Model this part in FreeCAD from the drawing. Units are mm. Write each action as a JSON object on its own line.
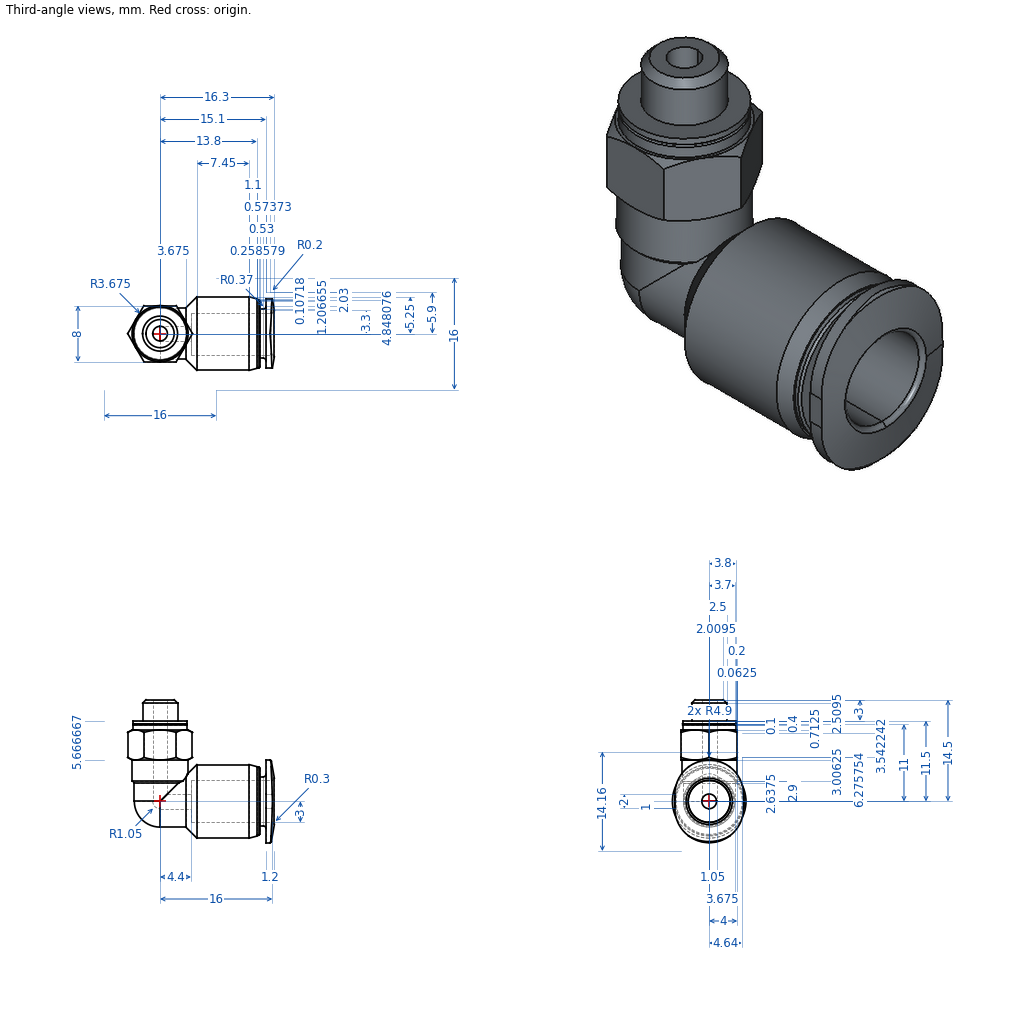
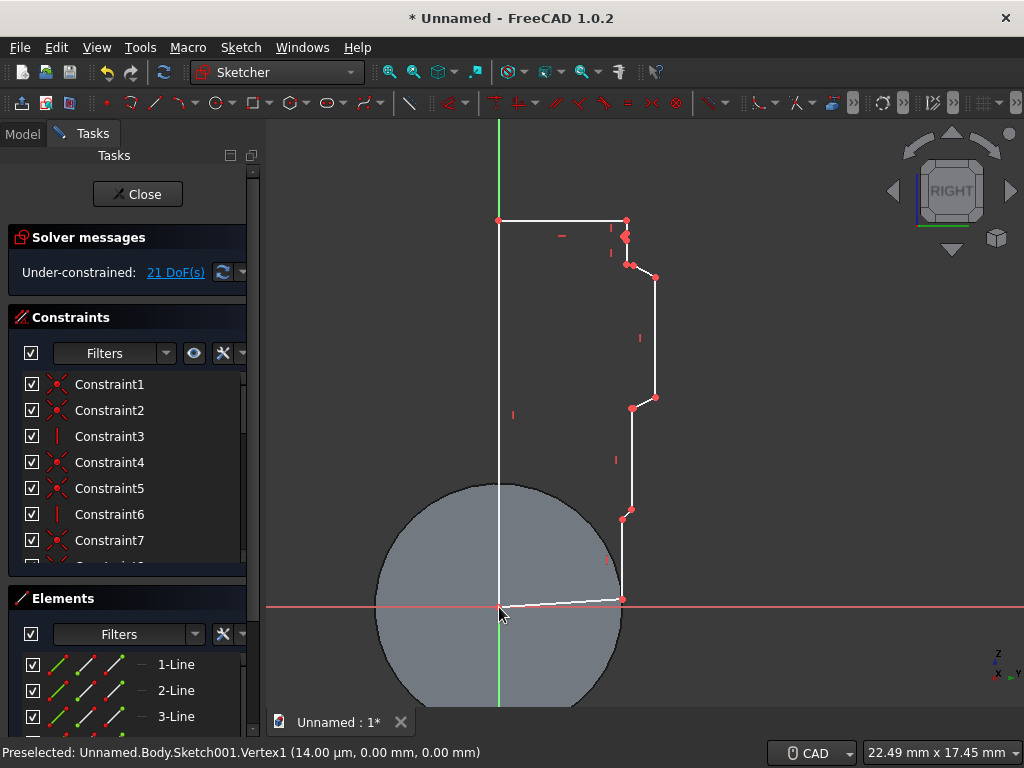
{"action": "left_click", "coordinate": [536, 605]}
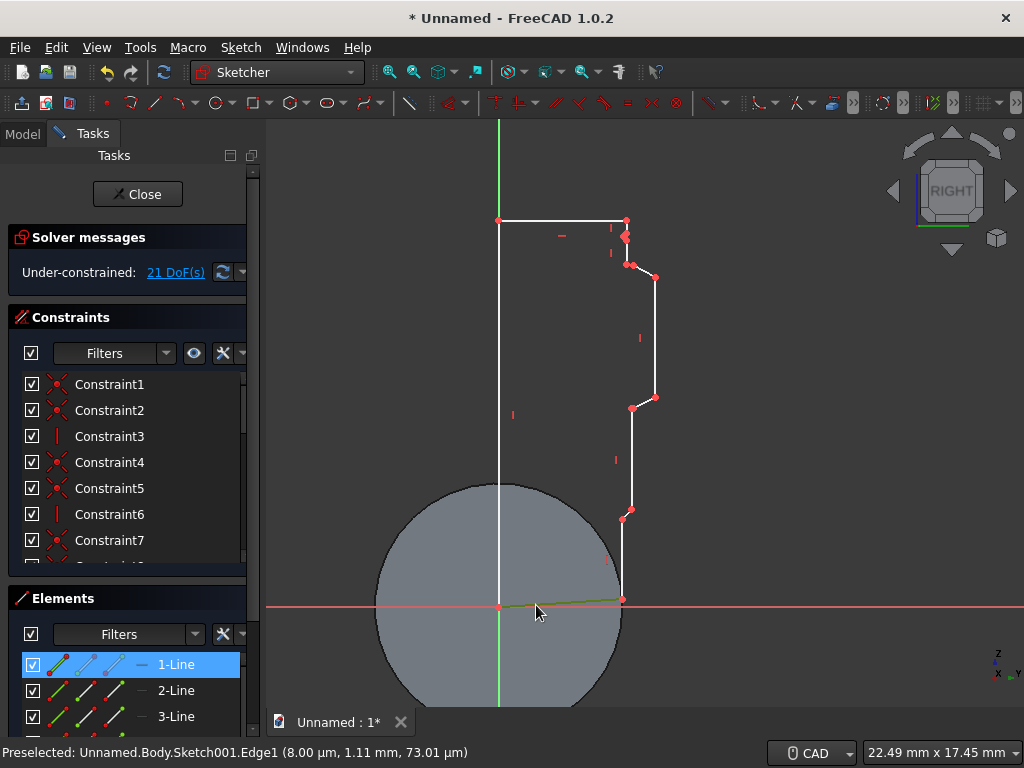
{"action": "key", "text": "h"}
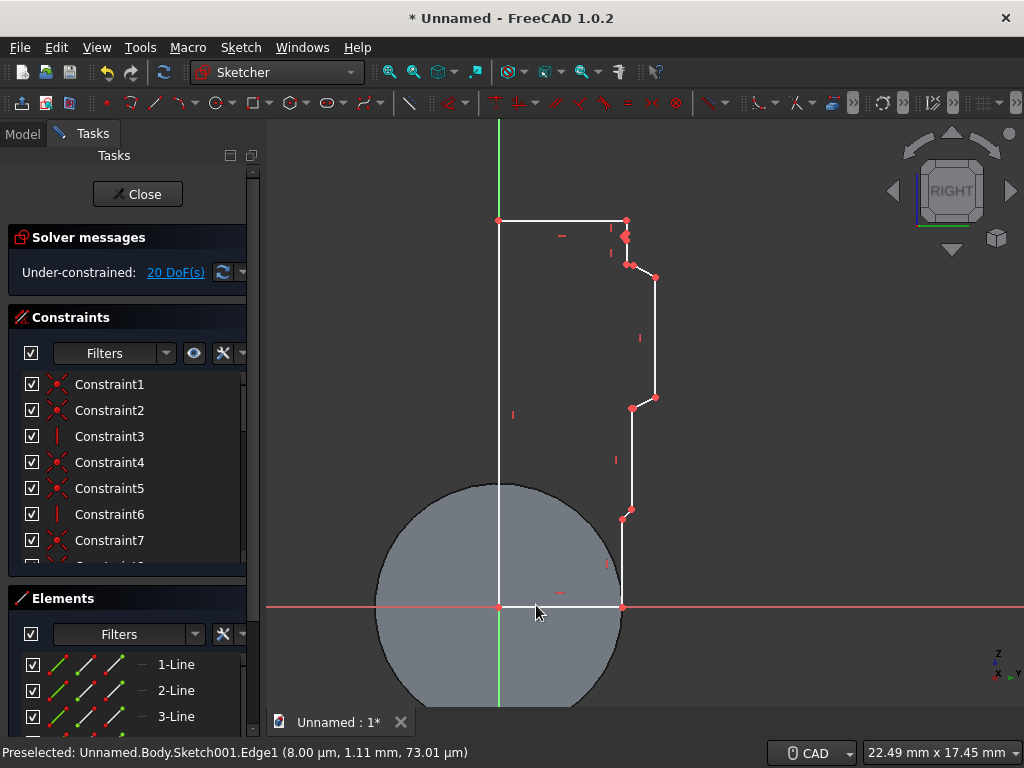
{"action": "scroll", "coordinate": [633, 408], "scroll_direction": "up", "scroll_amount": 14}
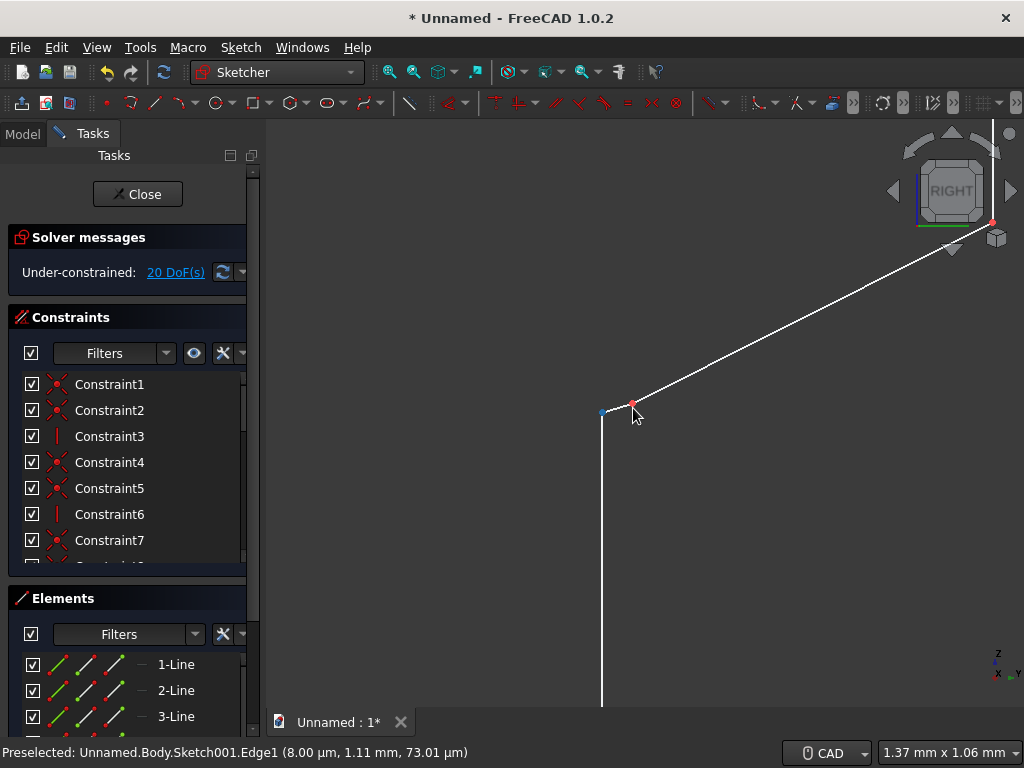
{"action": "left_click", "coordinate": [618, 408]}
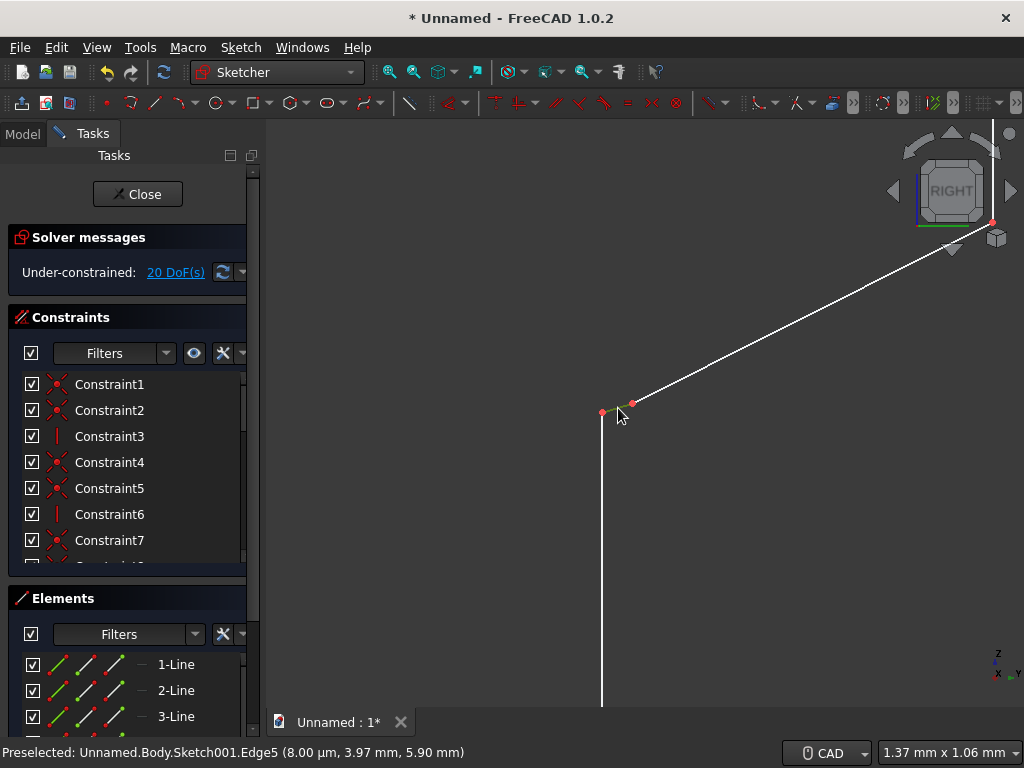
{"action": "left_click", "coordinate": [538, 104]}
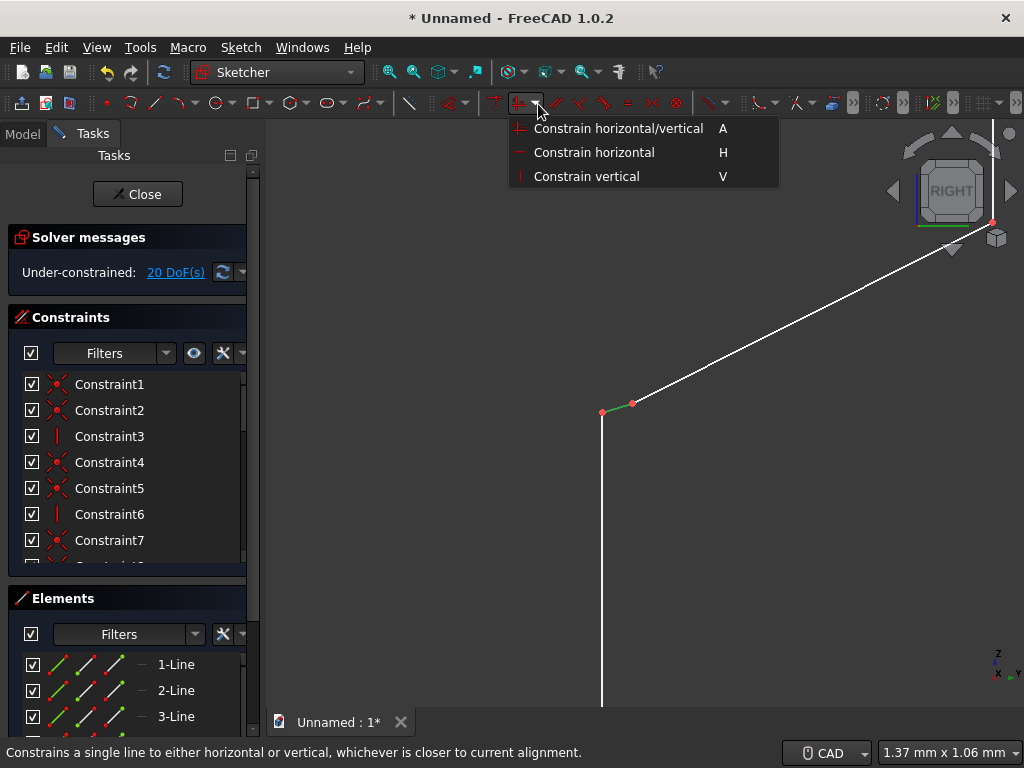
{"action": "left_click", "coordinate": [644, 152]}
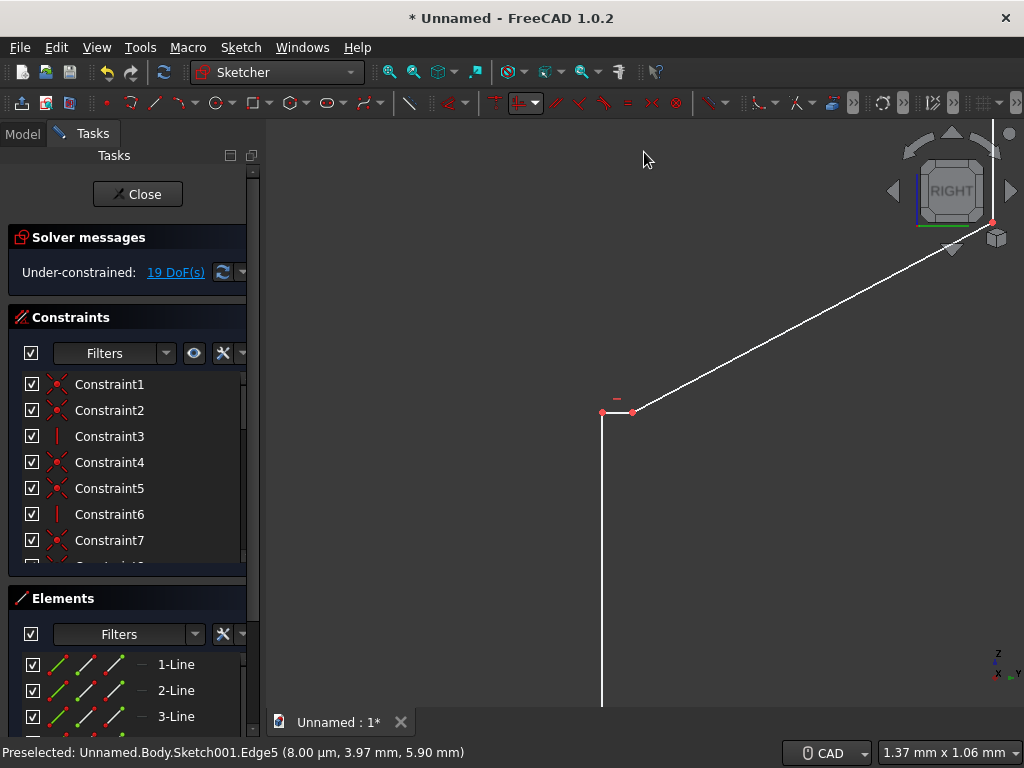
{"action": "scroll", "coordinate": [633, 408], "scroll_direction": "down", "scroll_amount": 14}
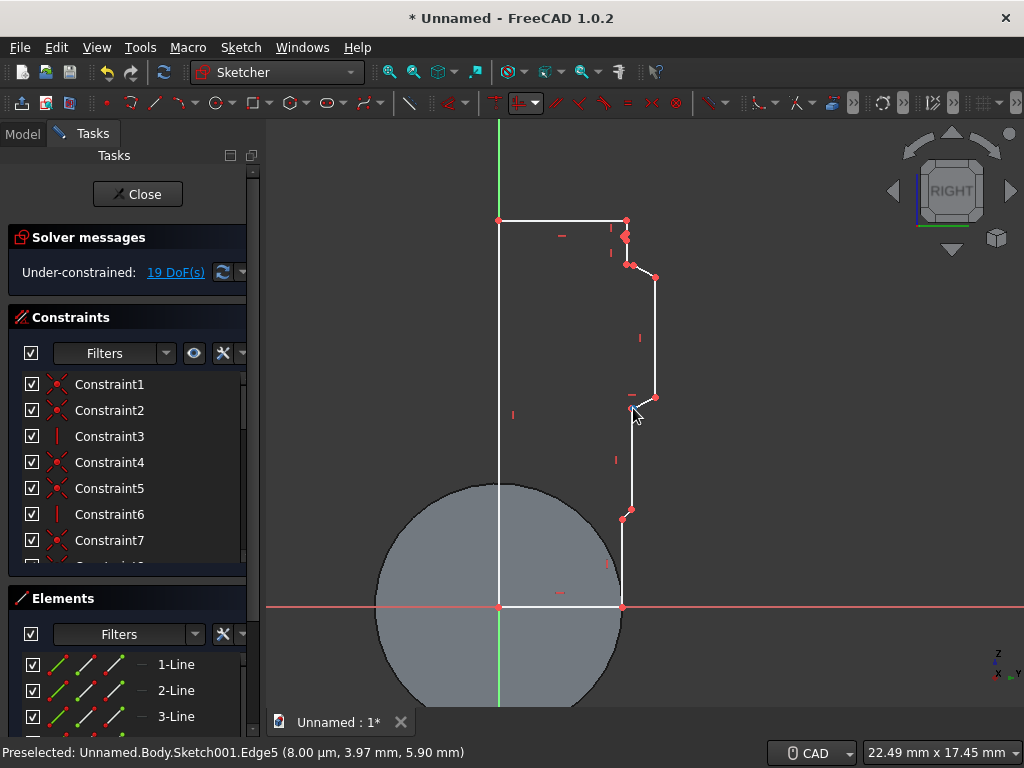
{"action": "scroll", "coordinate": [631, 265], "scroll_direction": "up", "scroll_amount": 10}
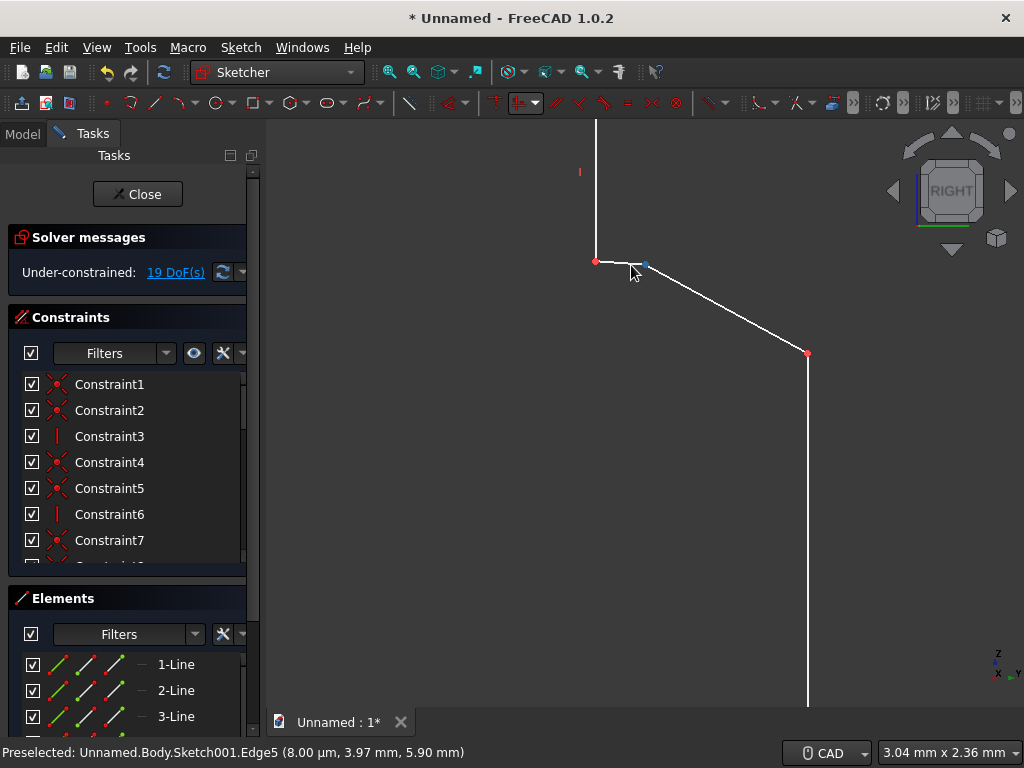
{"action": "left_click", "coordinate": [630, 264]}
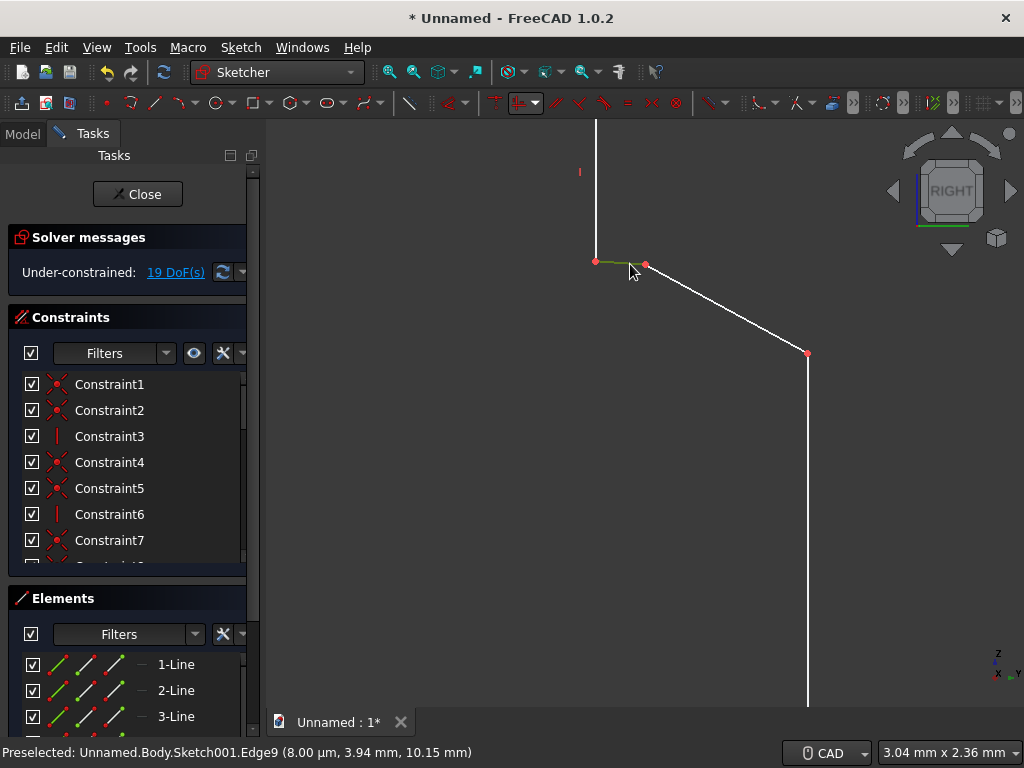
{"action": "left_click", "coordinate": [538, 104]}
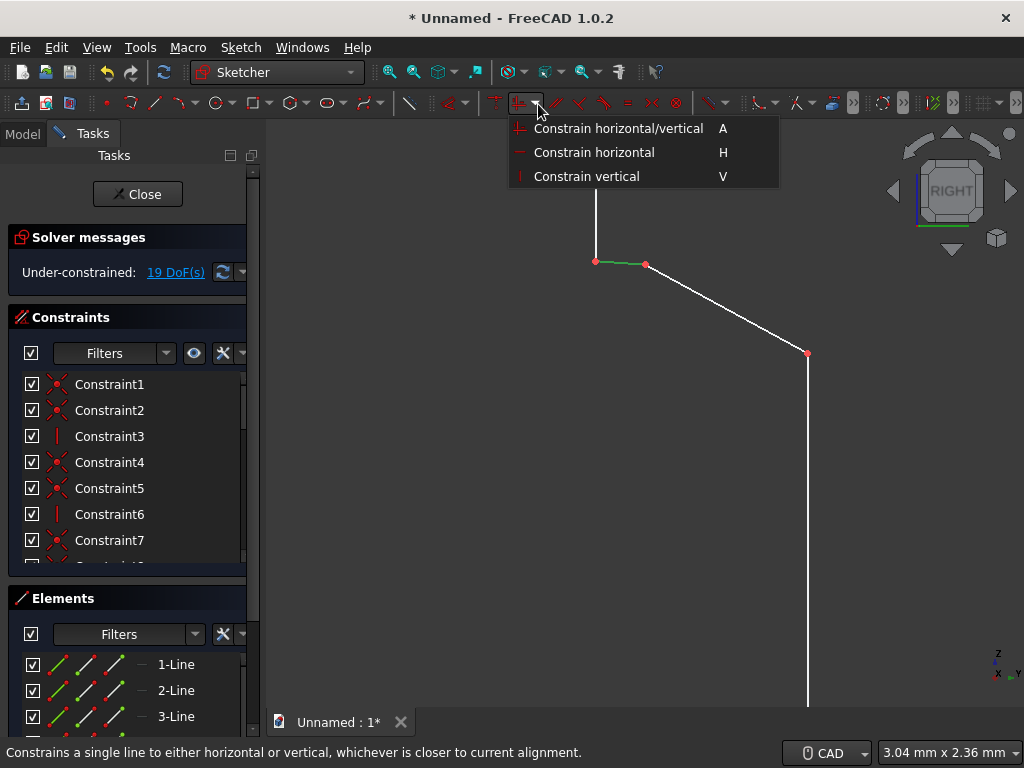
{"action": "left_click", "coordinate": [644, 152]}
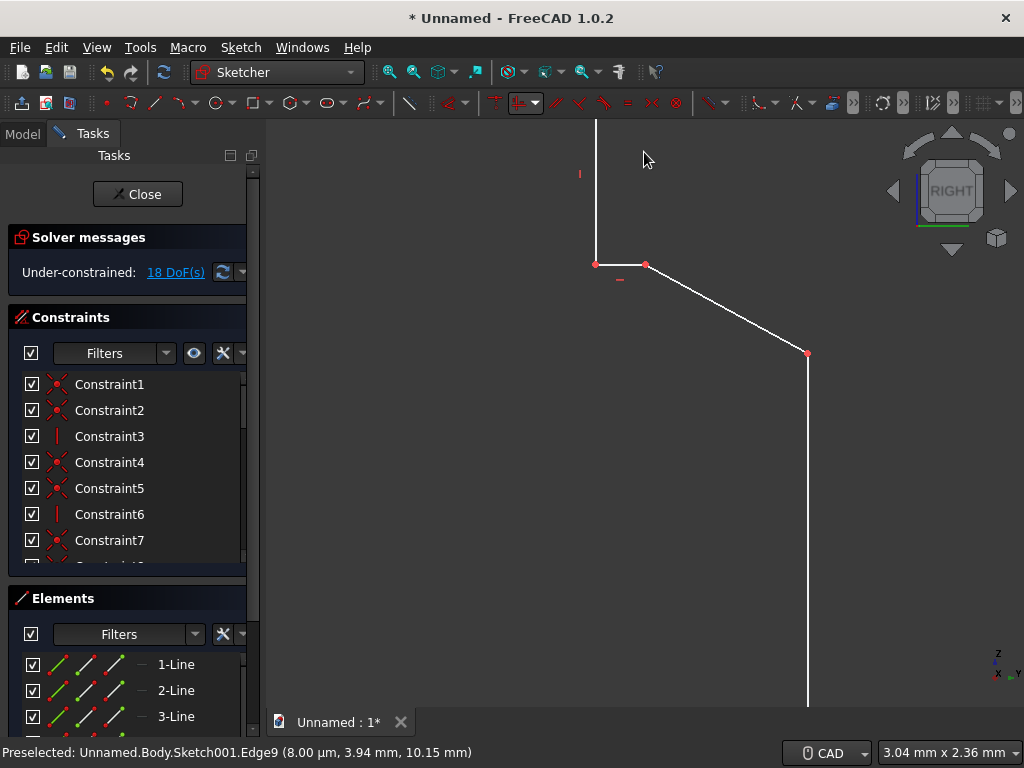
{"action": "left_click", "coordinate": [448, 104]}